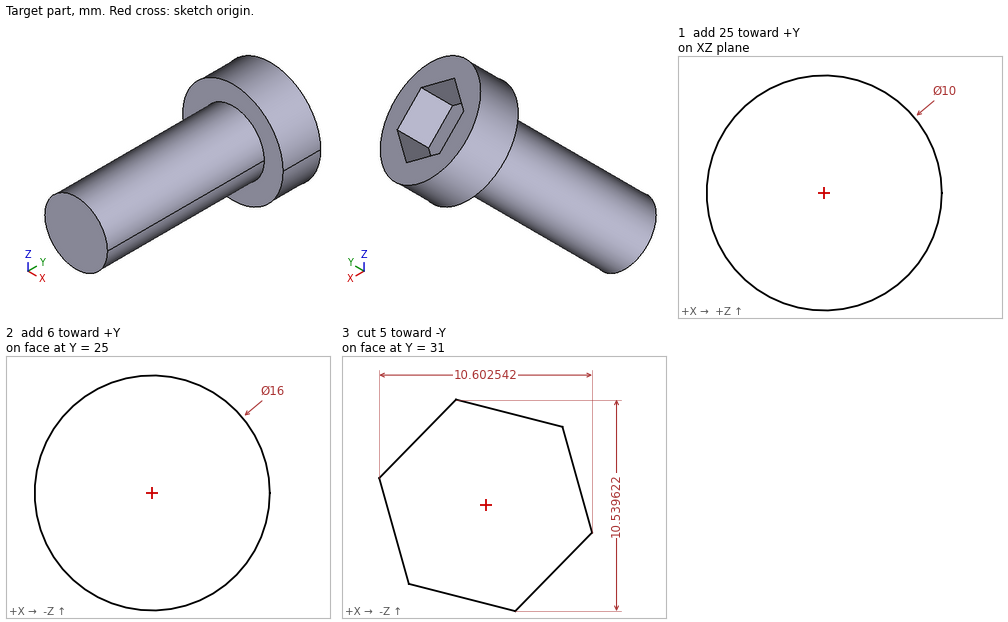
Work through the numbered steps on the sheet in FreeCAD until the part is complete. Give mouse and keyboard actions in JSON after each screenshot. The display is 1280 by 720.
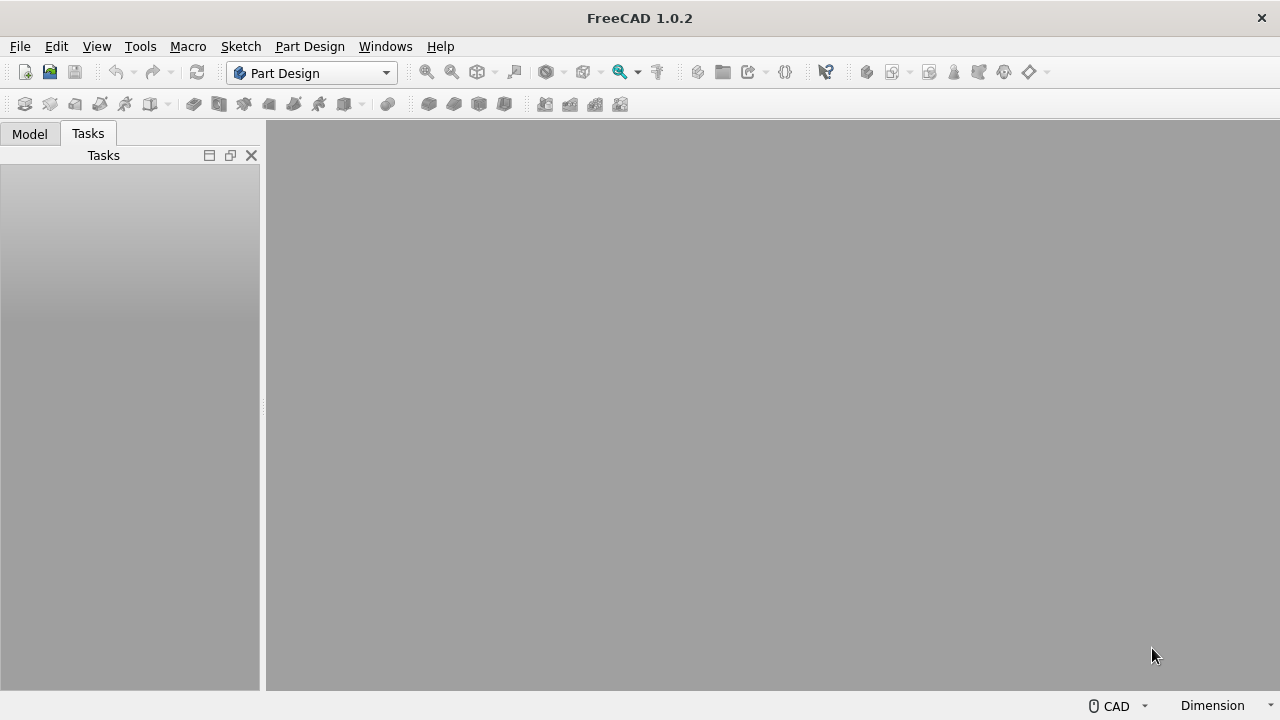
{"action": "key", "text": "ctrl+n"}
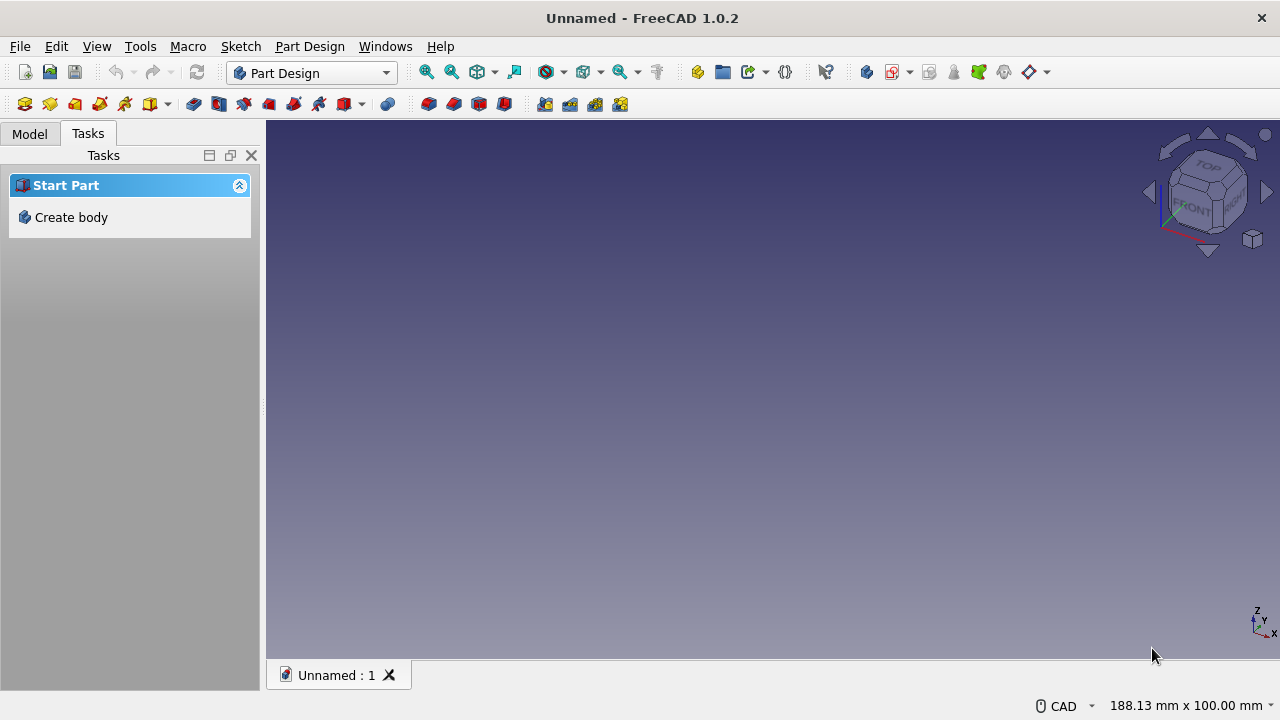
{"action": "left_click", "coordinate": [892, 72]}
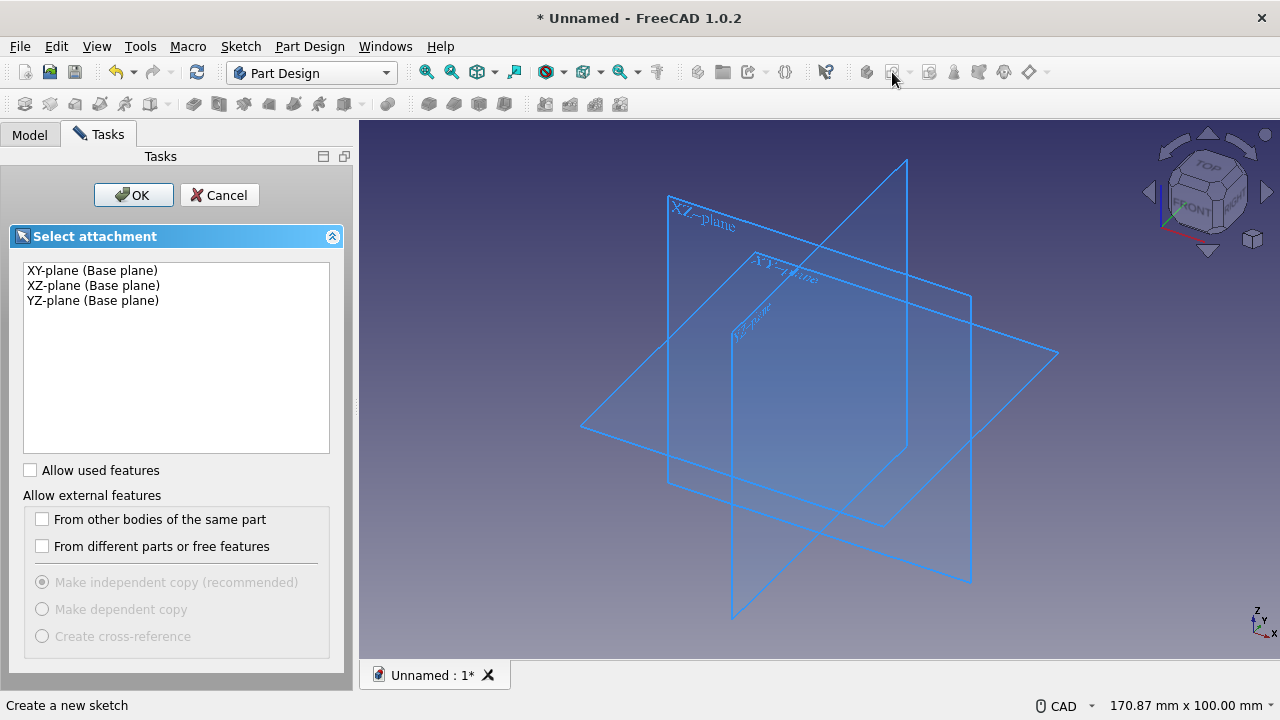
{"action": "left_click", "coordinate": [84, 286]}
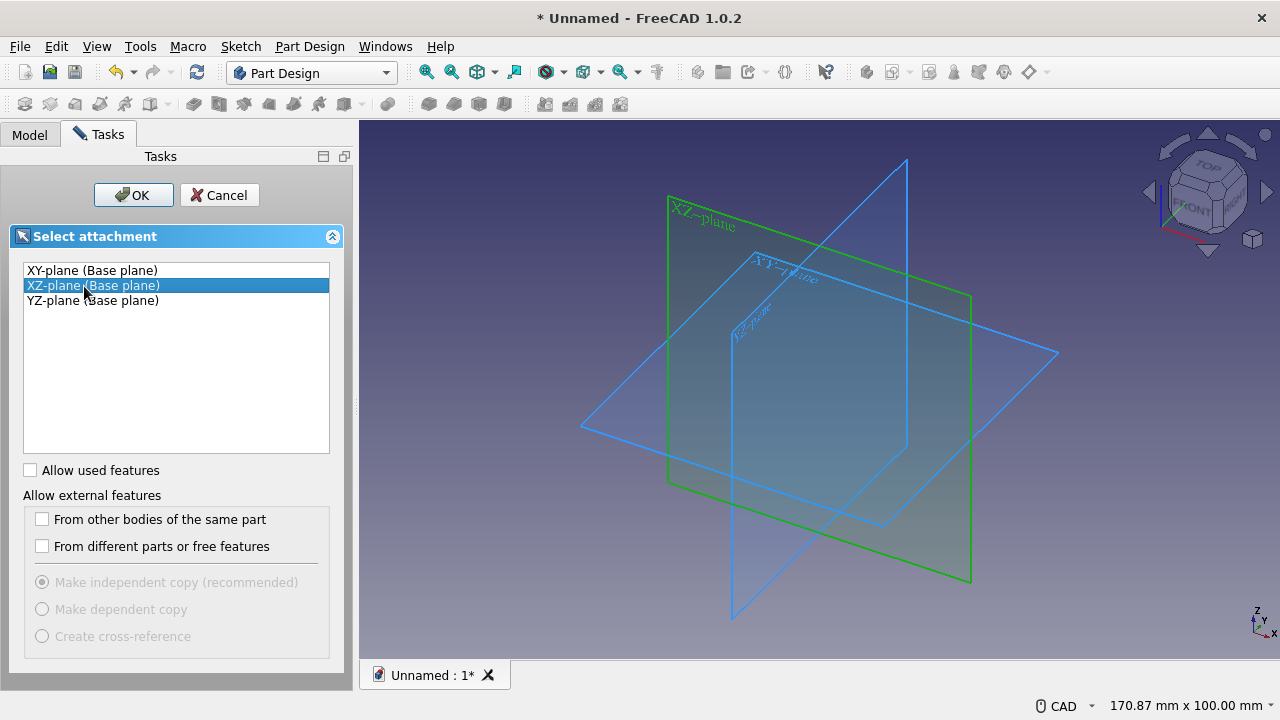
{"action": "left_click", "coordinate": [134, 195]}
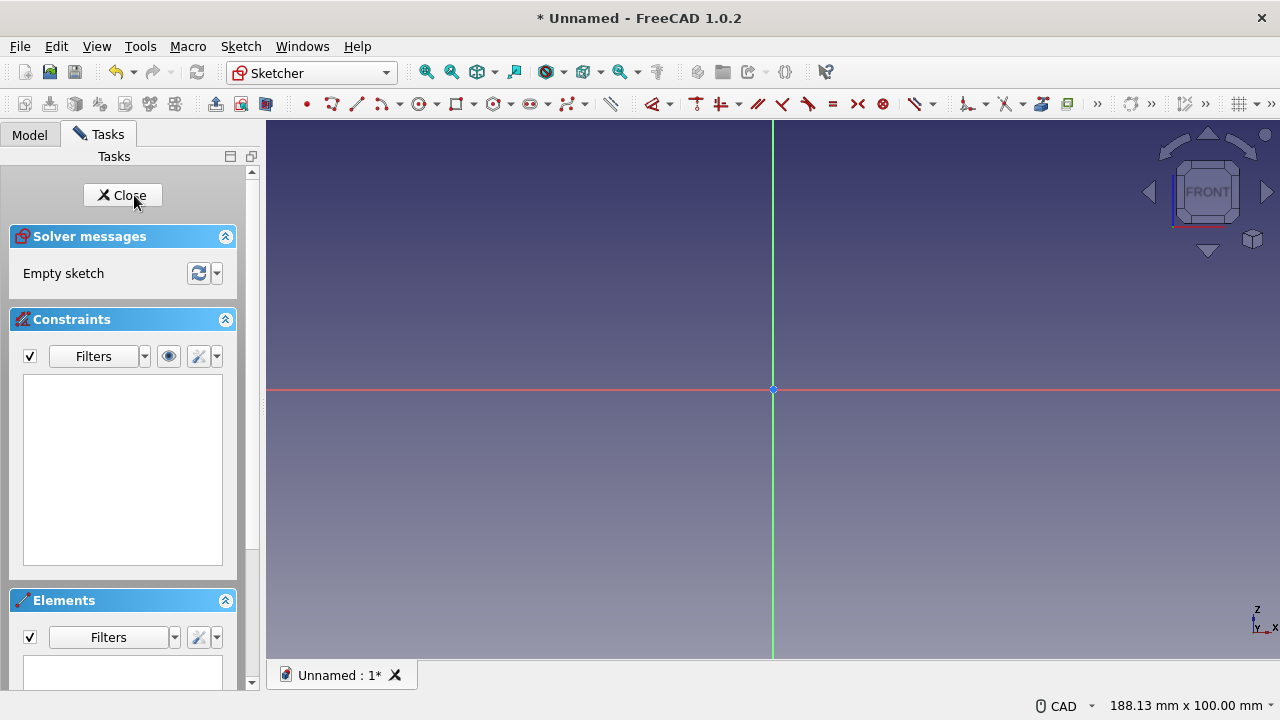
{"action": "scroll", "coordinate": [787, 390], "scroll_direction": "up", "scroll_amount": 9}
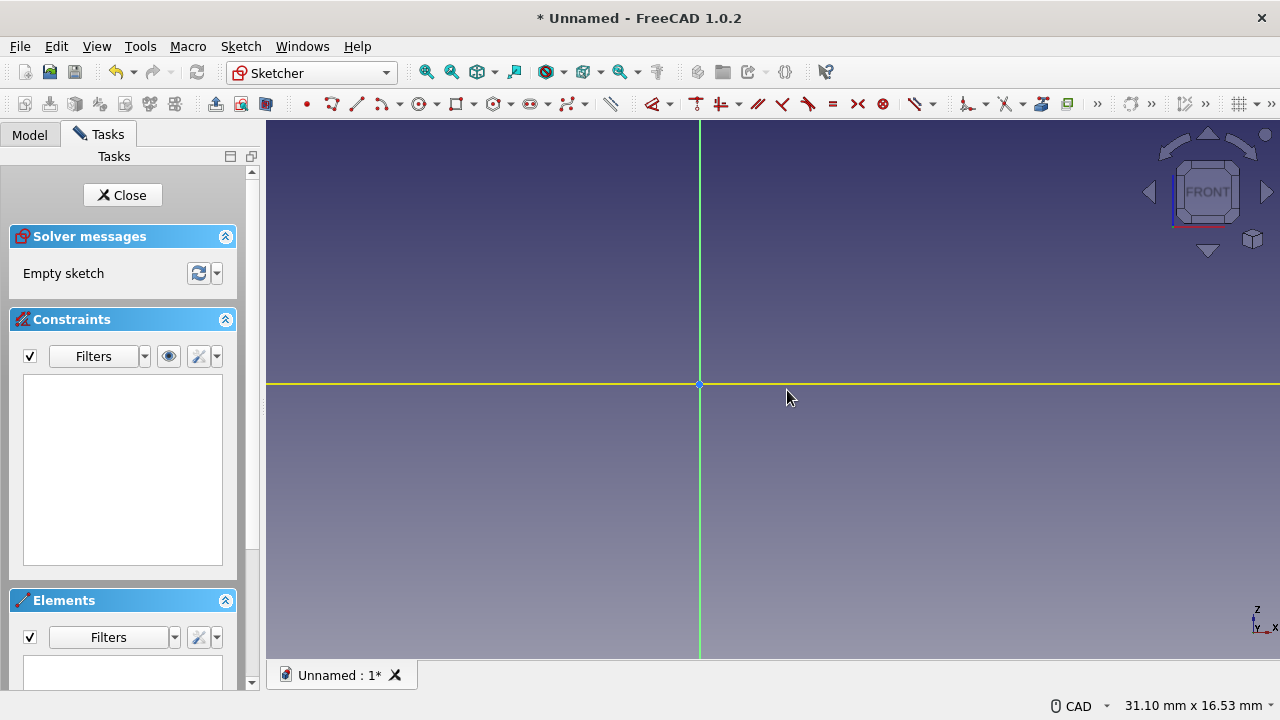
{"action": "key", "text": "g c"}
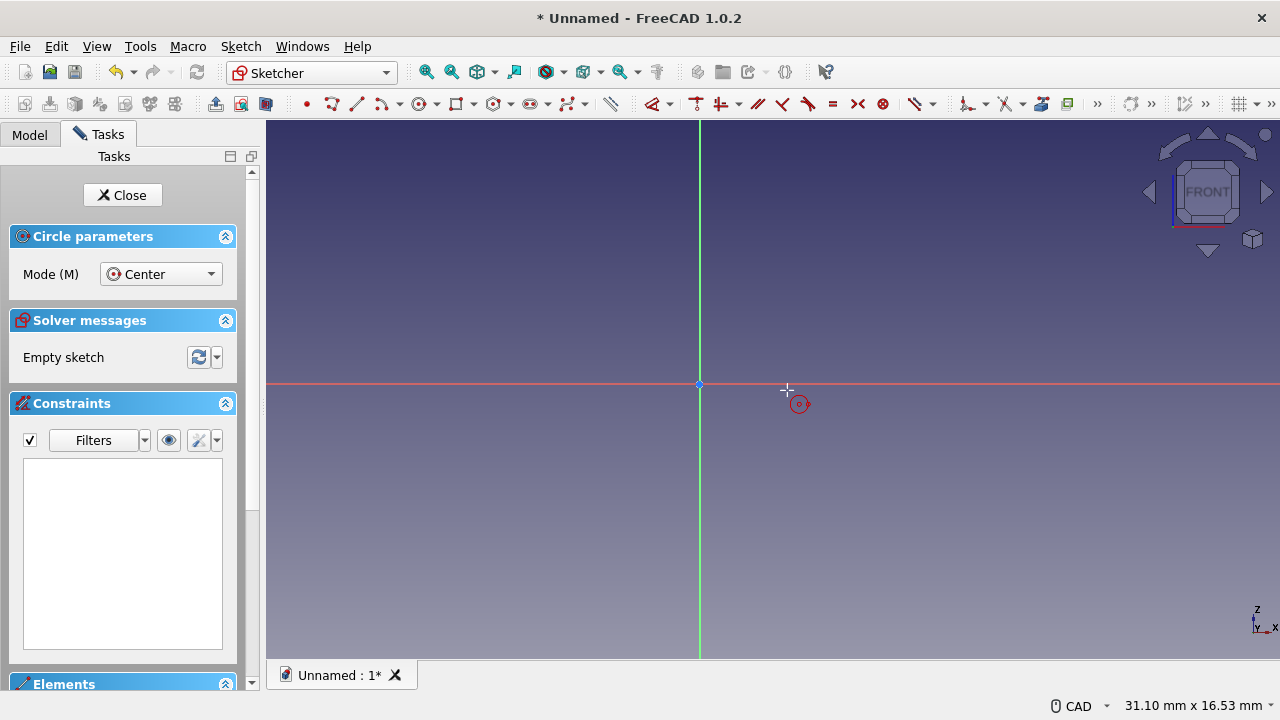
{"action": "left_click", "coordinate": [700, 384]}
{"action": "mouse_move", "coordinate": [815, 269]}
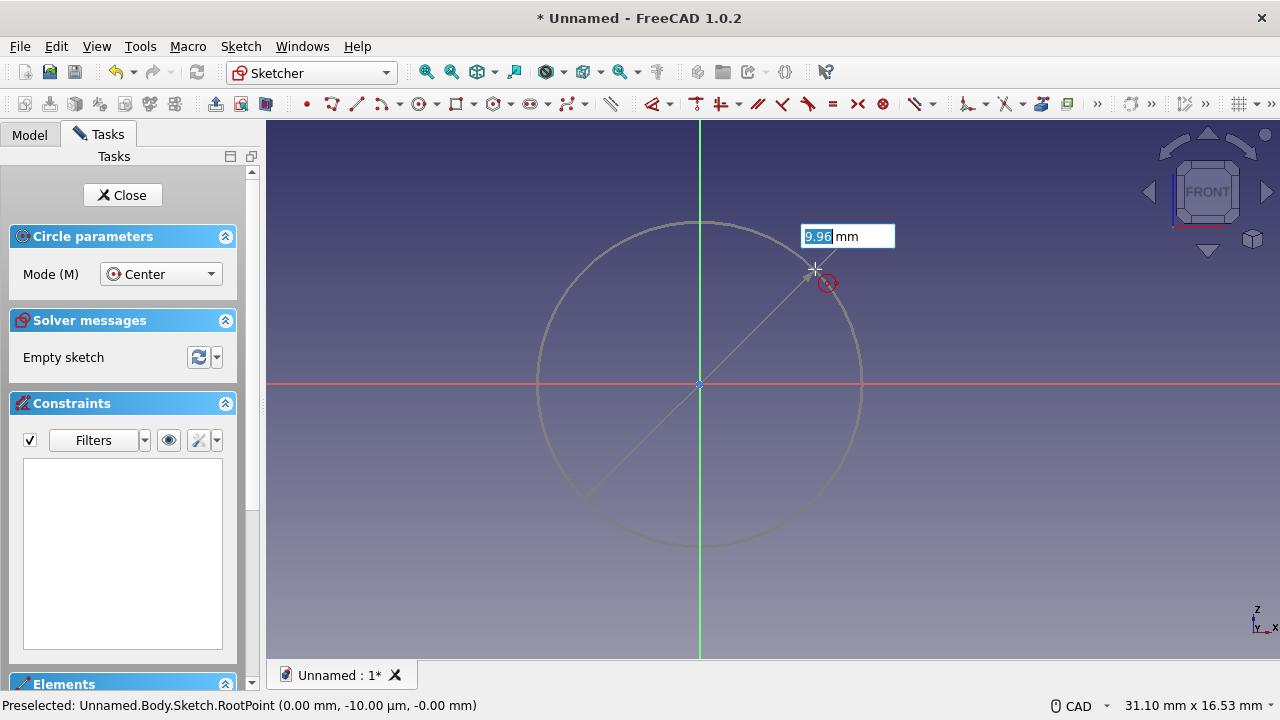
{"action": "type", "text": "10"}
{"action": "key", "text": "Return"}
{"action": "key", "text": "Escape"}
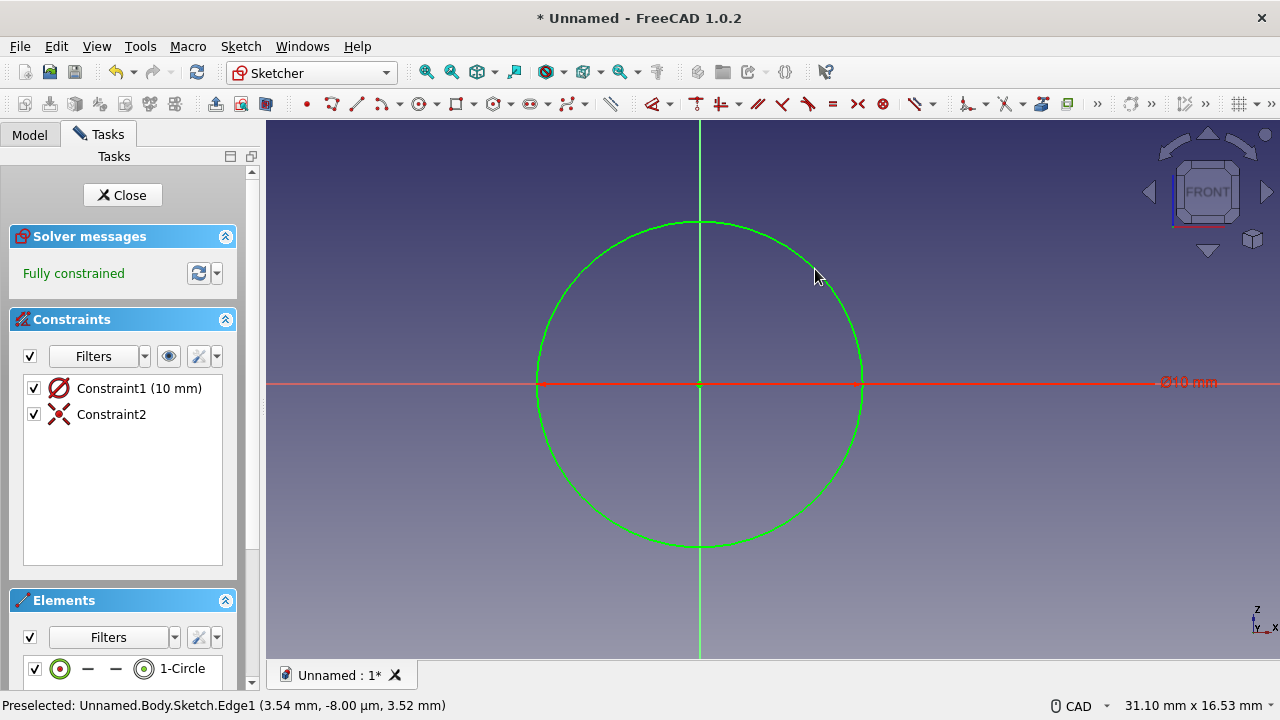
{"action": "left_click", "coordinate": [123, 195]}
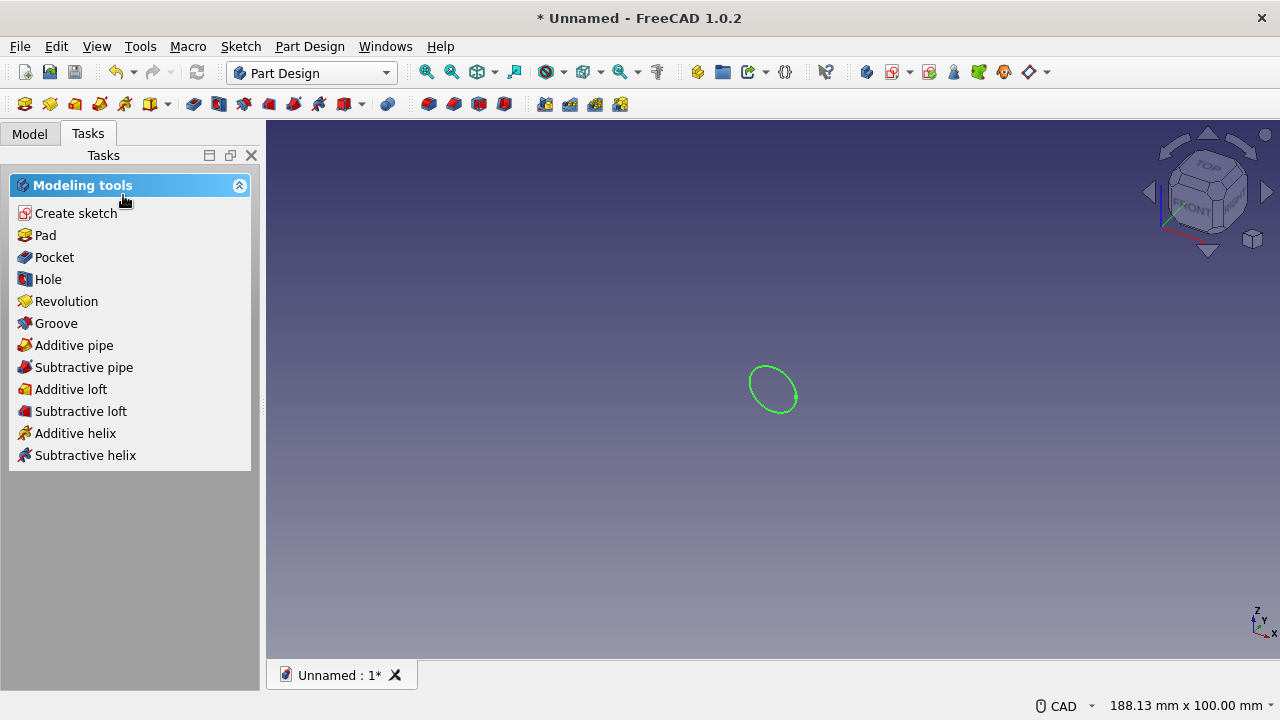
{"action": "left_click", "coordinate": [25, 104]}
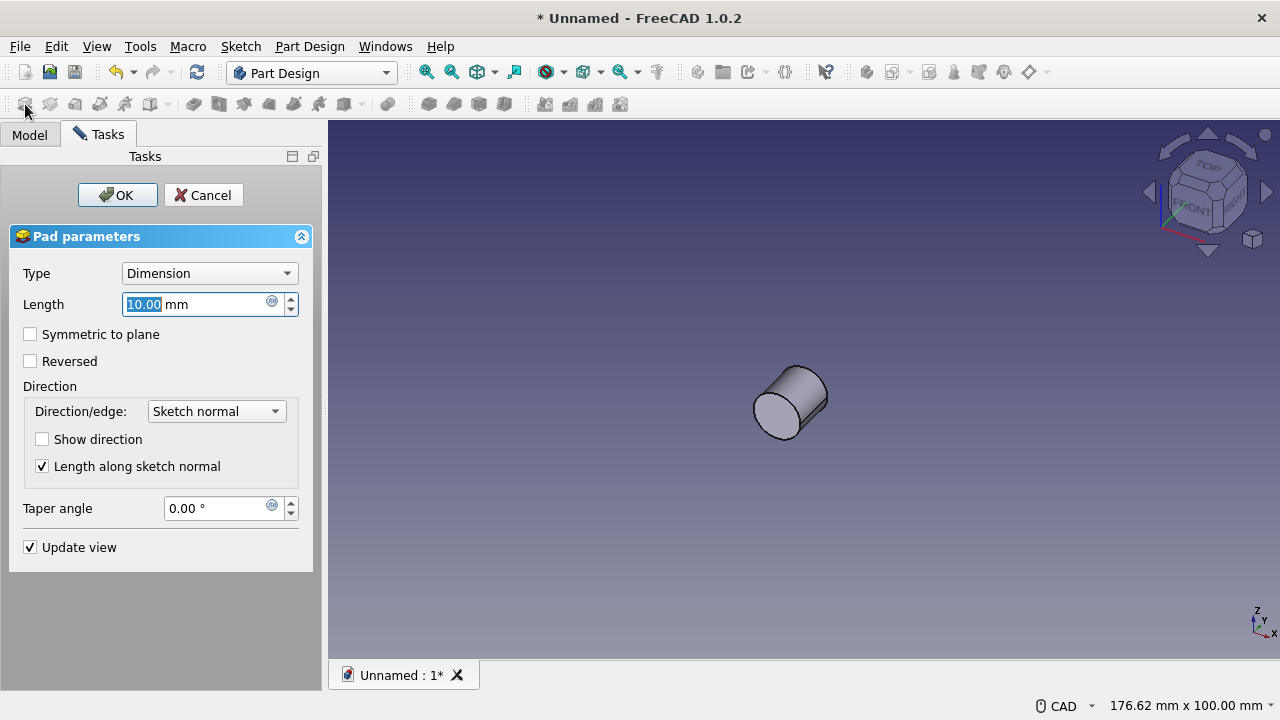
{"action": "type", "text": "25"}
{"action": "key", "text": "Tab"}